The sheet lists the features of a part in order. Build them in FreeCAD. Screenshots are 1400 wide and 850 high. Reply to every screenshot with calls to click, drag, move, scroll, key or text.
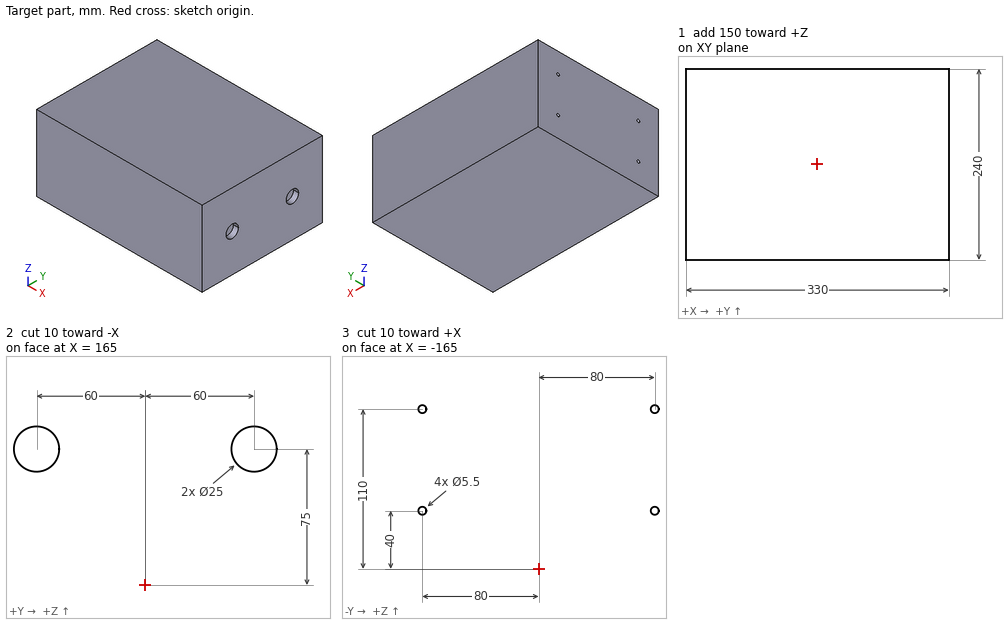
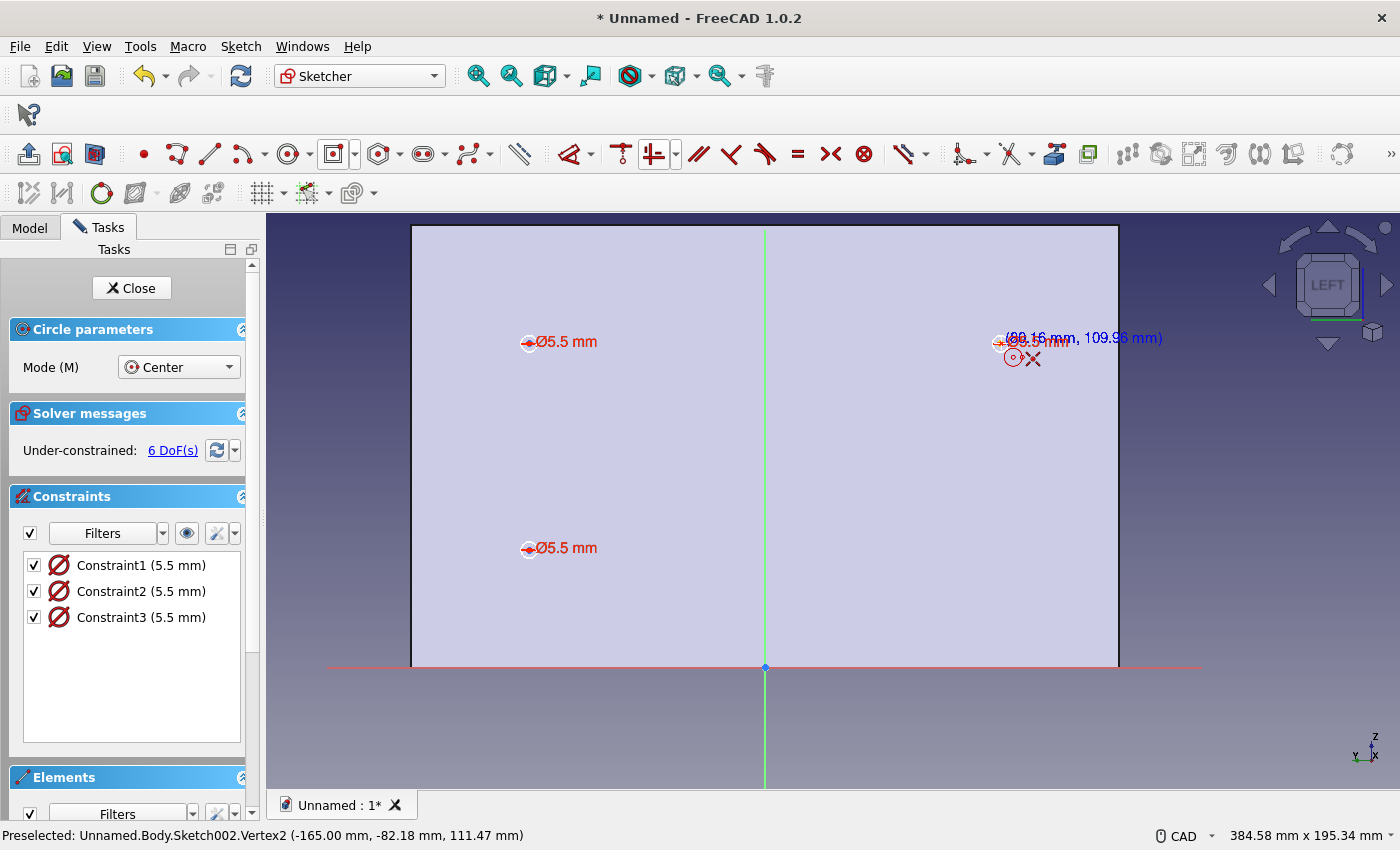
scroll(1001, 550, up, 6)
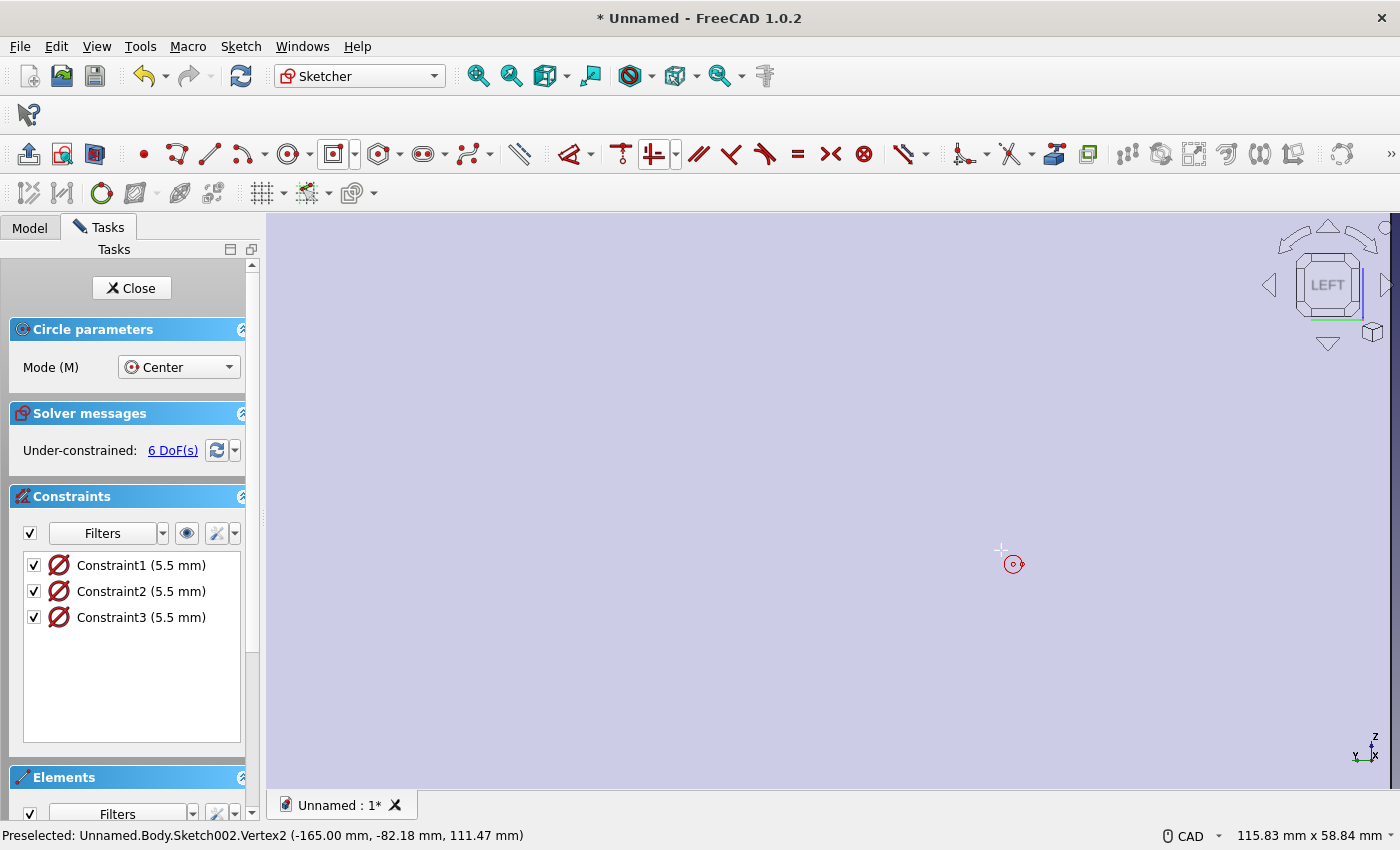
click(999, 548)
move(1018, 529)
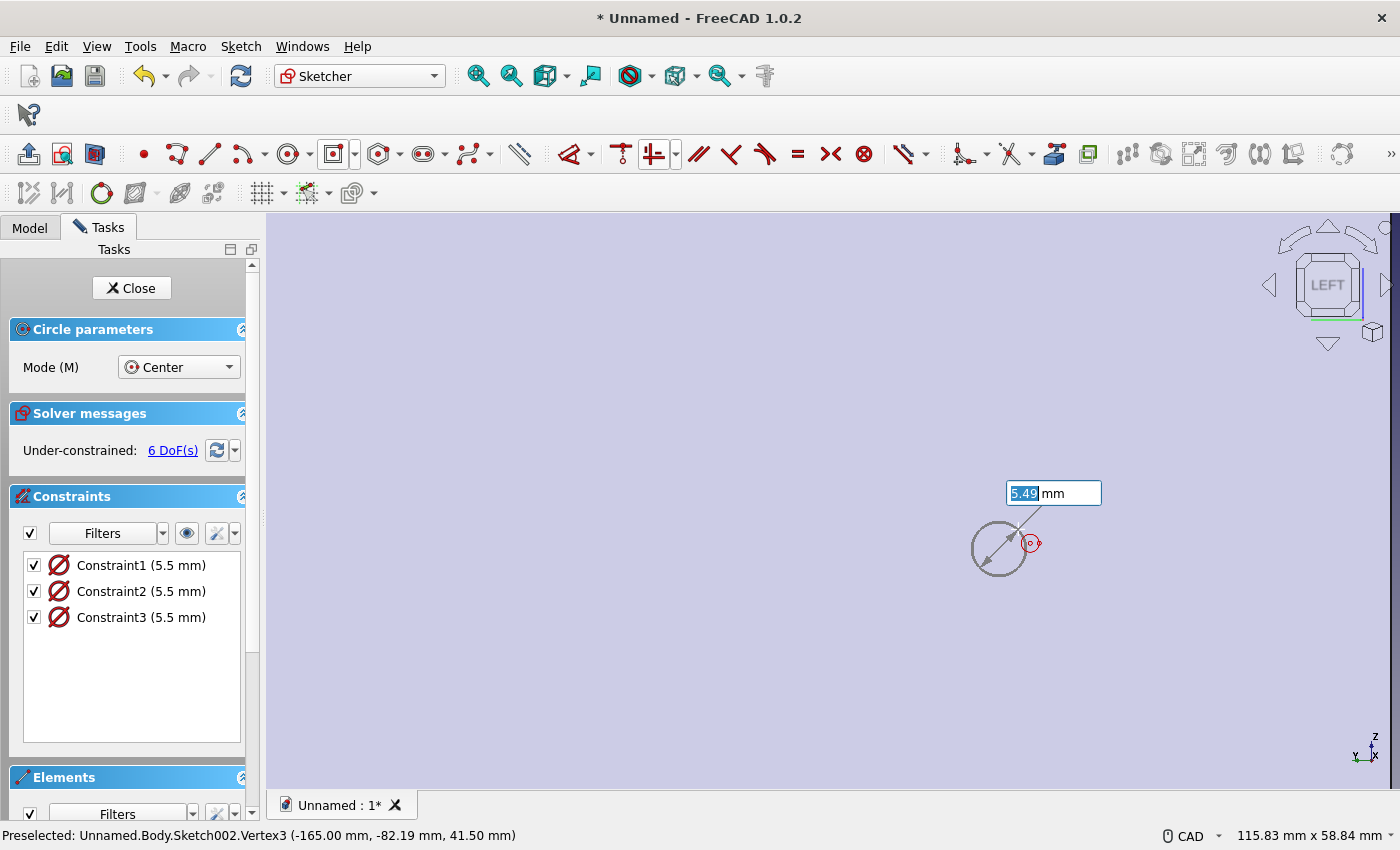
text(5.5)
key(Return)
key(Escape)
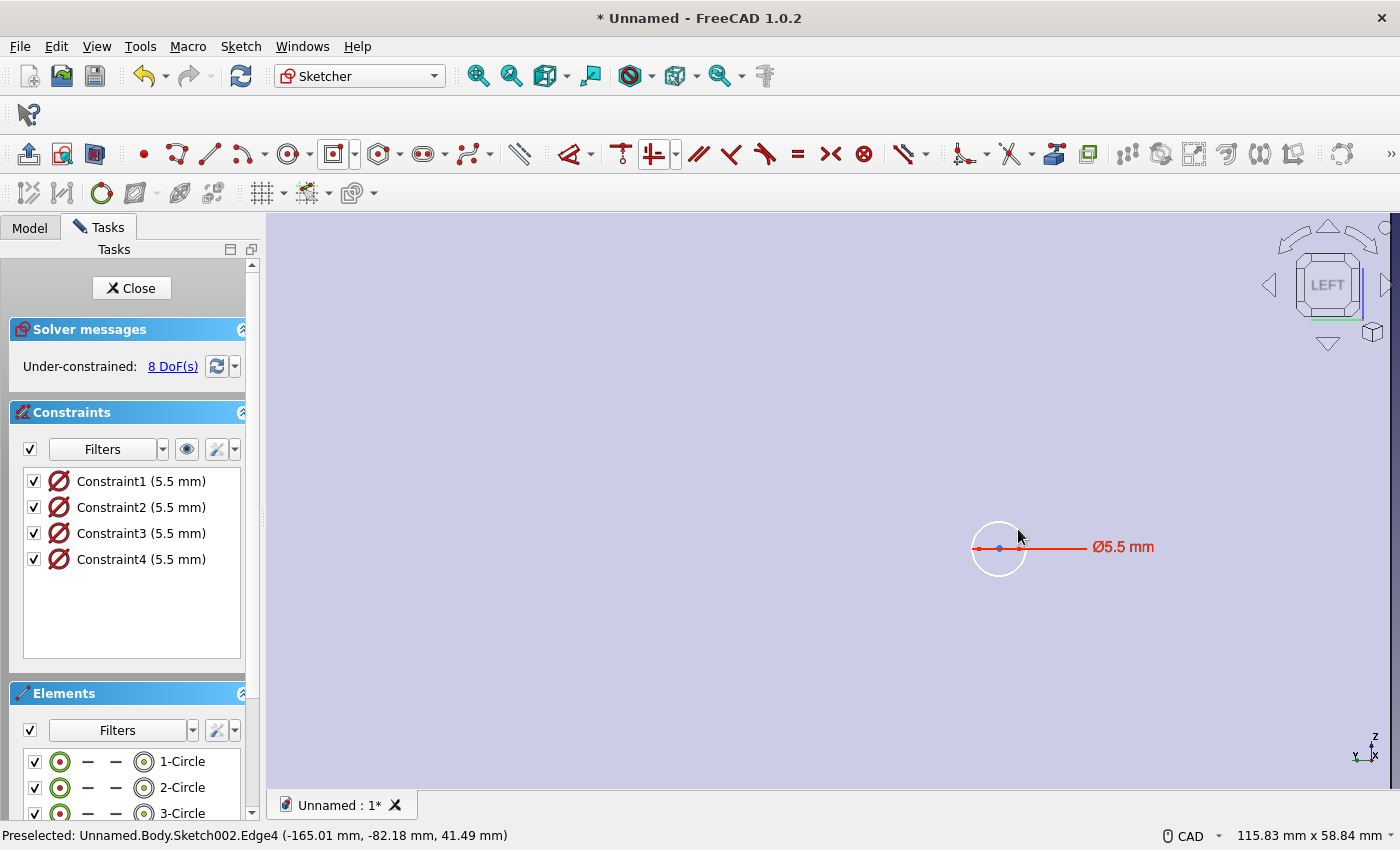
scroll(1001, 550, down, 6)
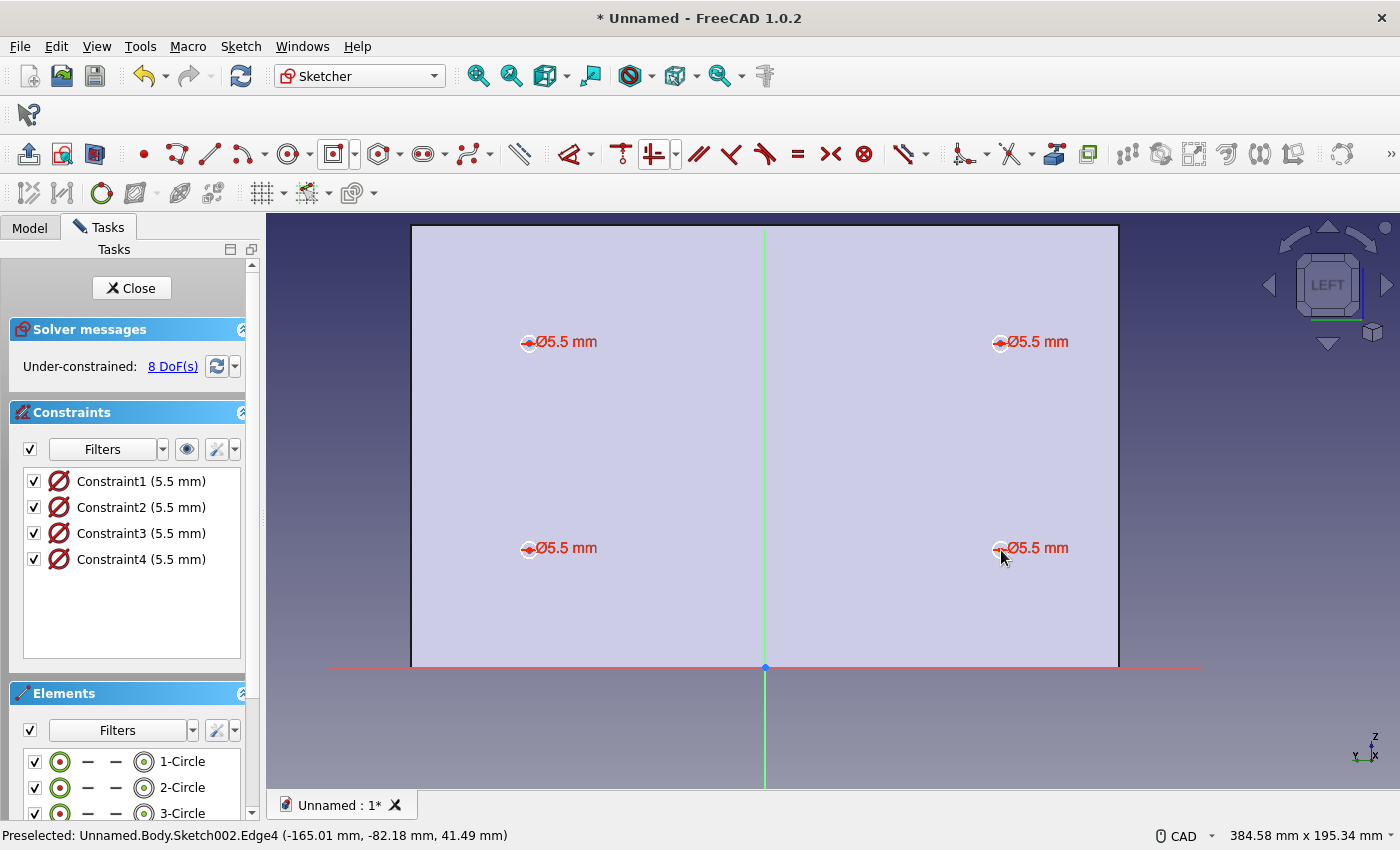
click(529, 550)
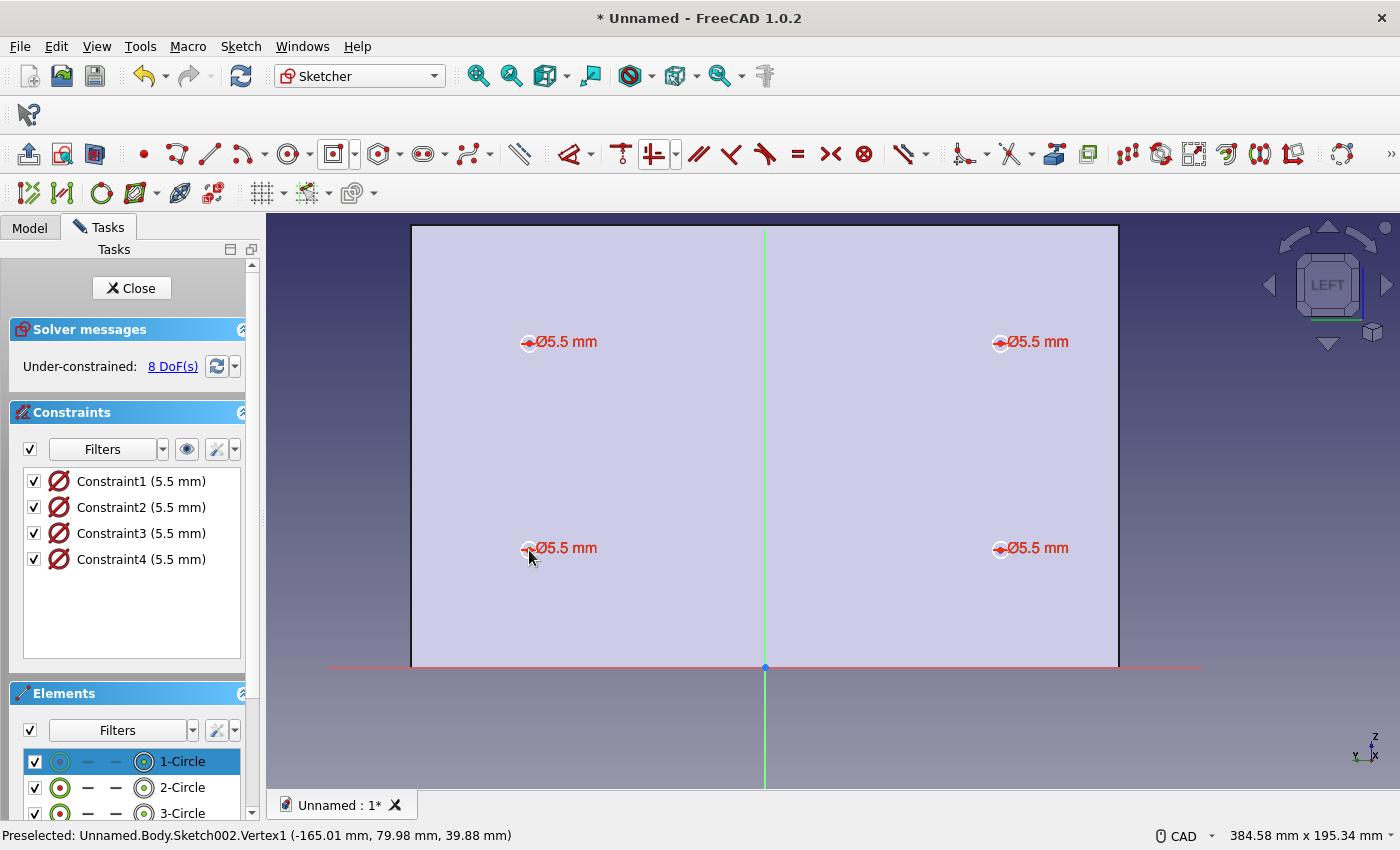
click(529, 344)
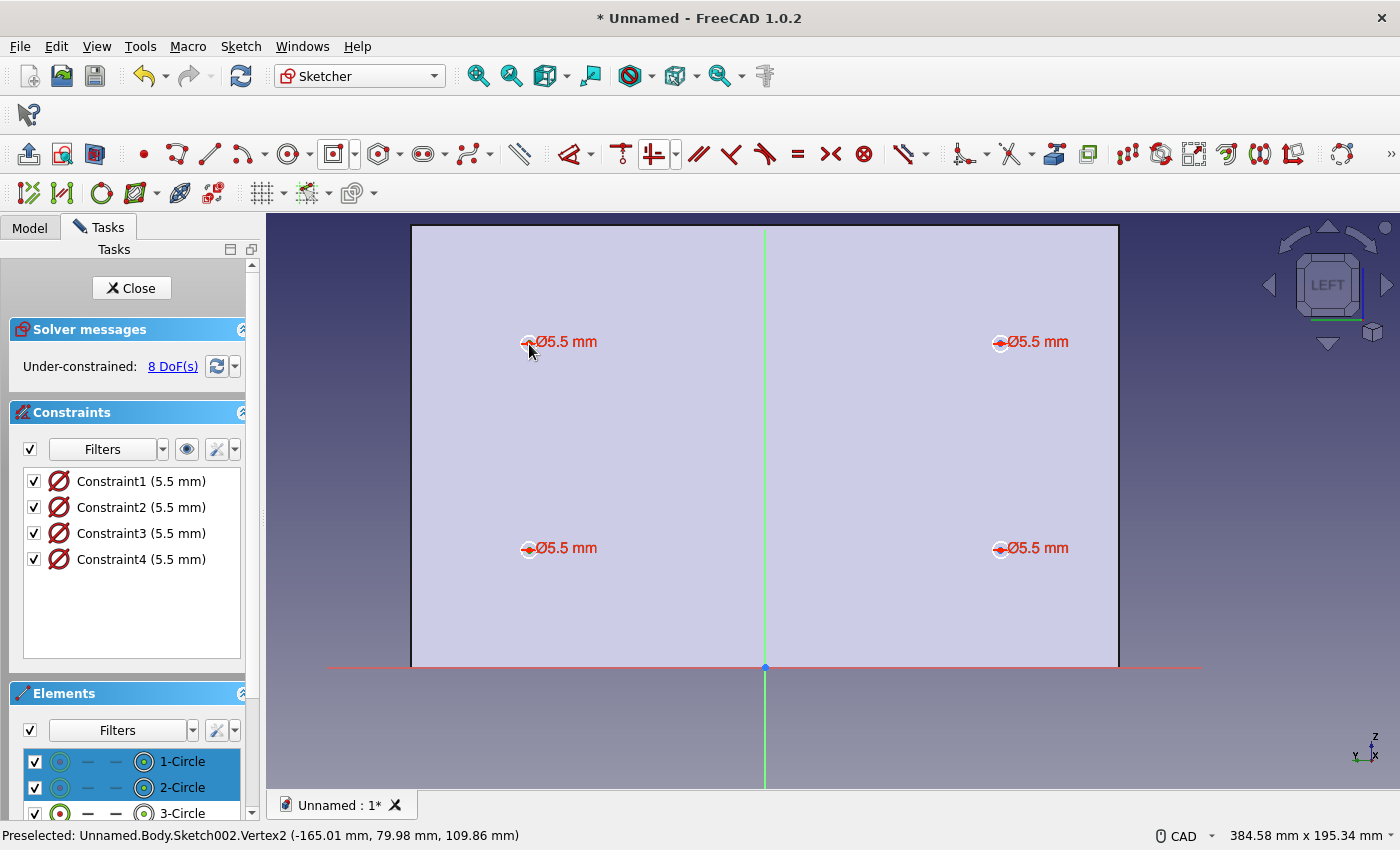
key(v)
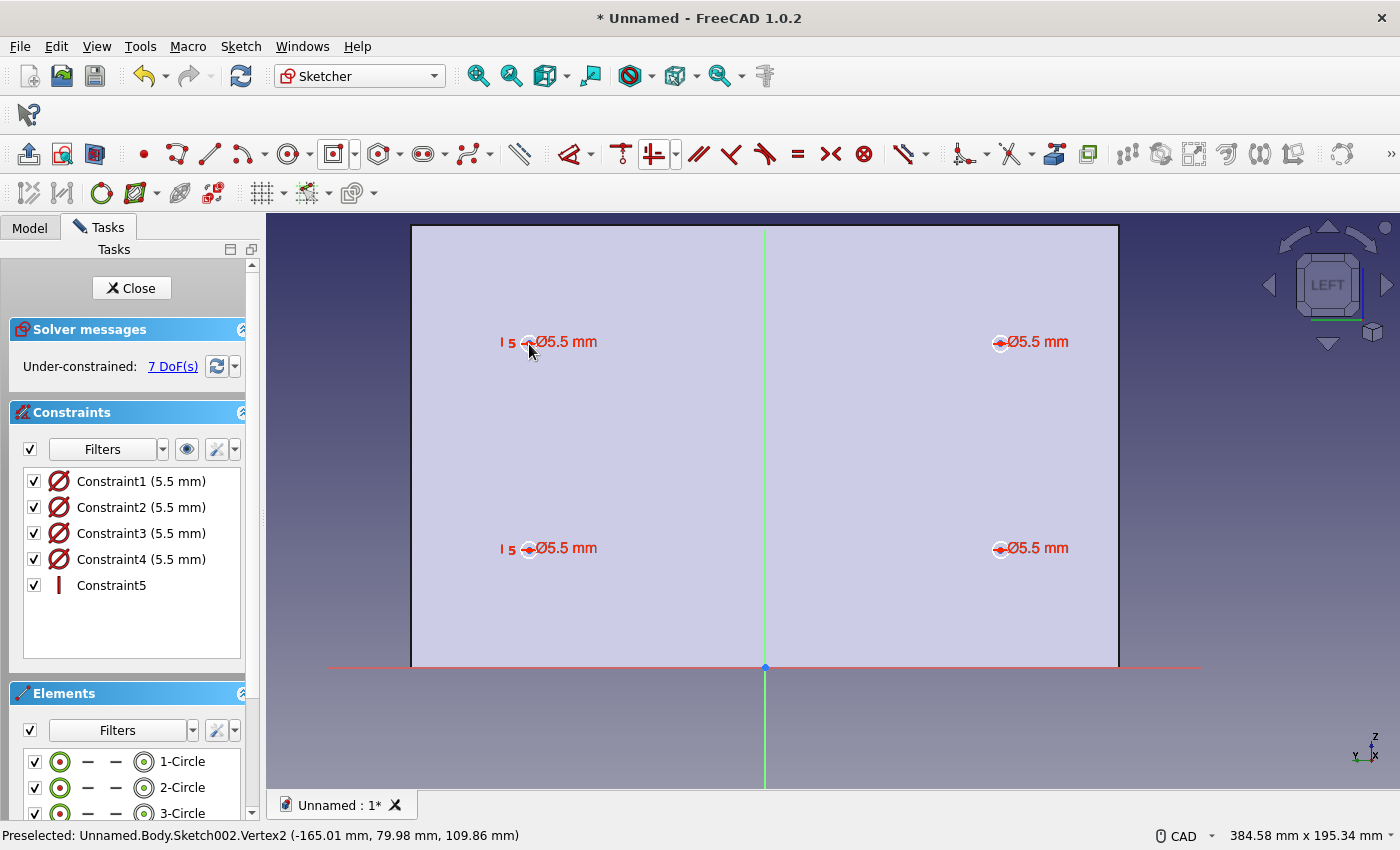
click(529, 344)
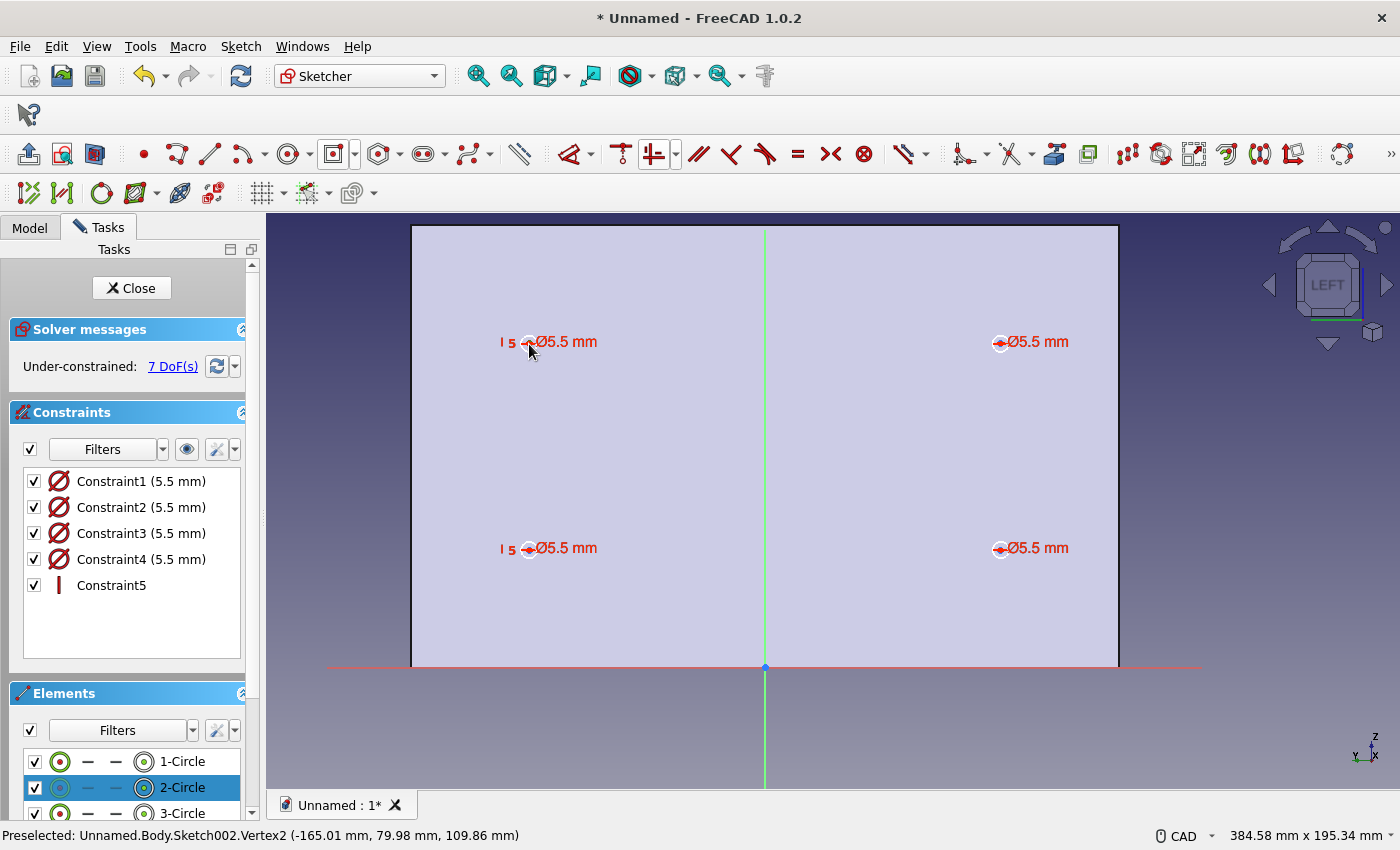
click(1001, 344)